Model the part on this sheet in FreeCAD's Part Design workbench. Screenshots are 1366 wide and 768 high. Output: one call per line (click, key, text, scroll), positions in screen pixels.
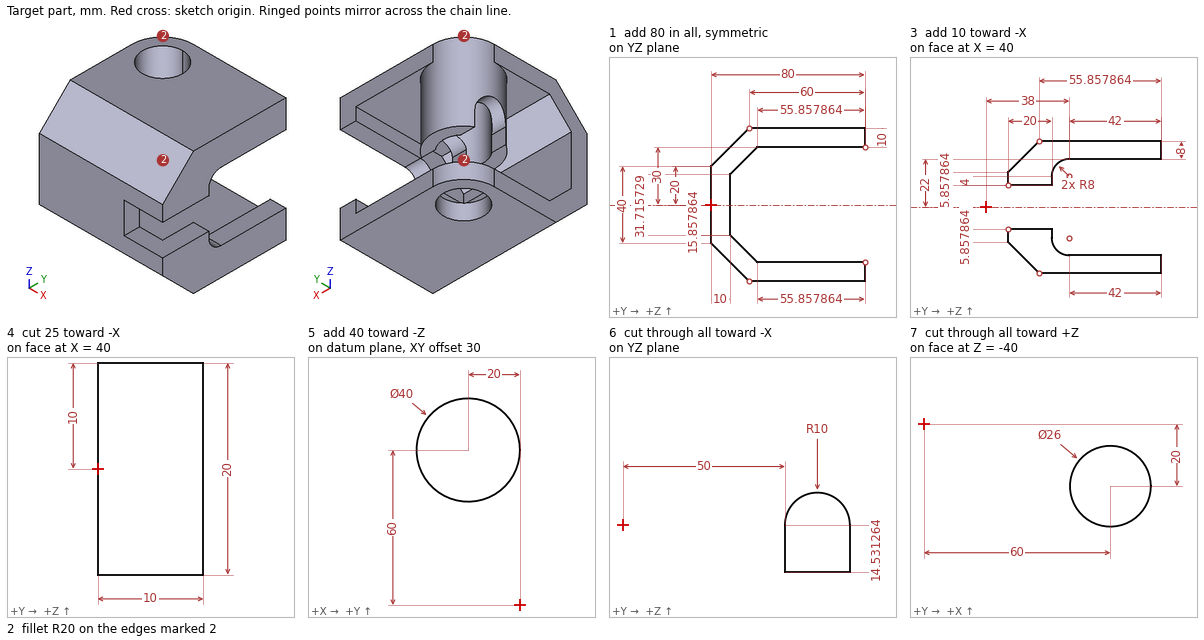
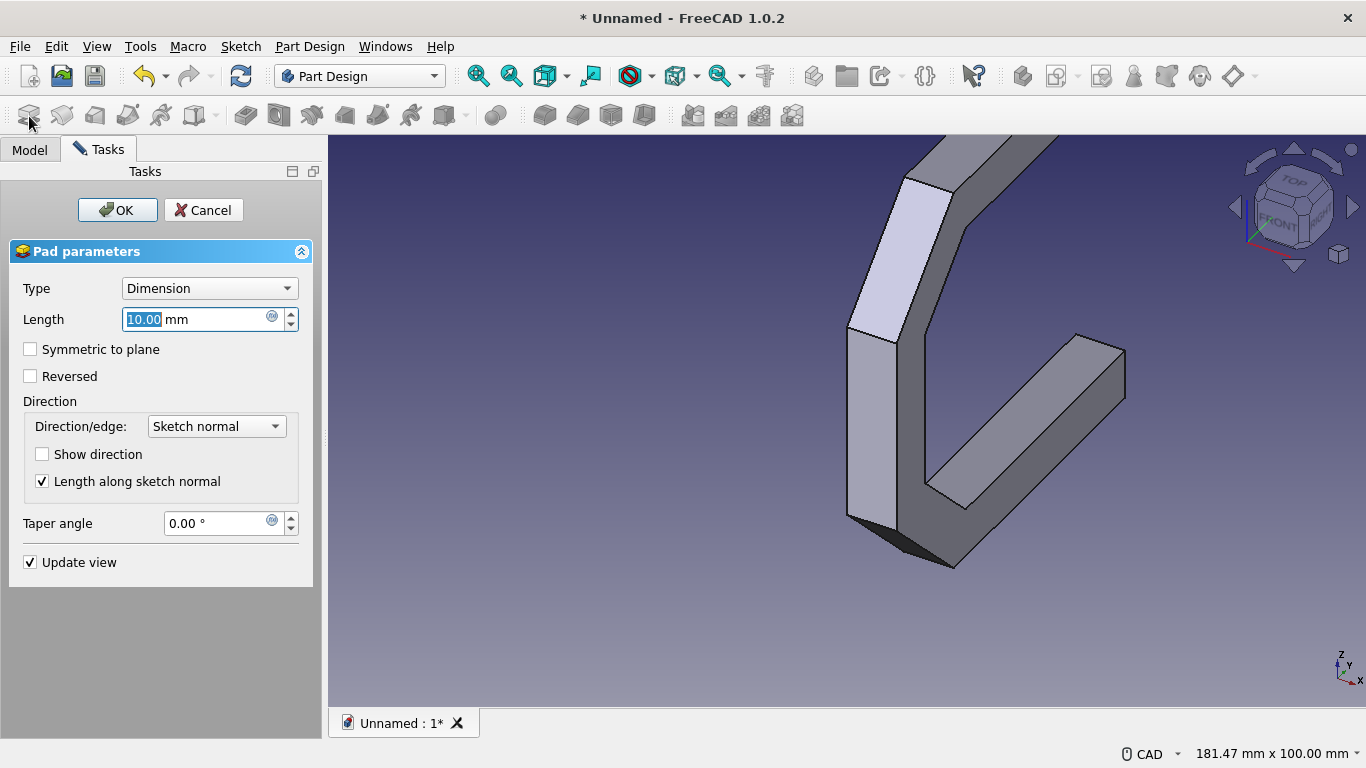
text(80)
key(Tab)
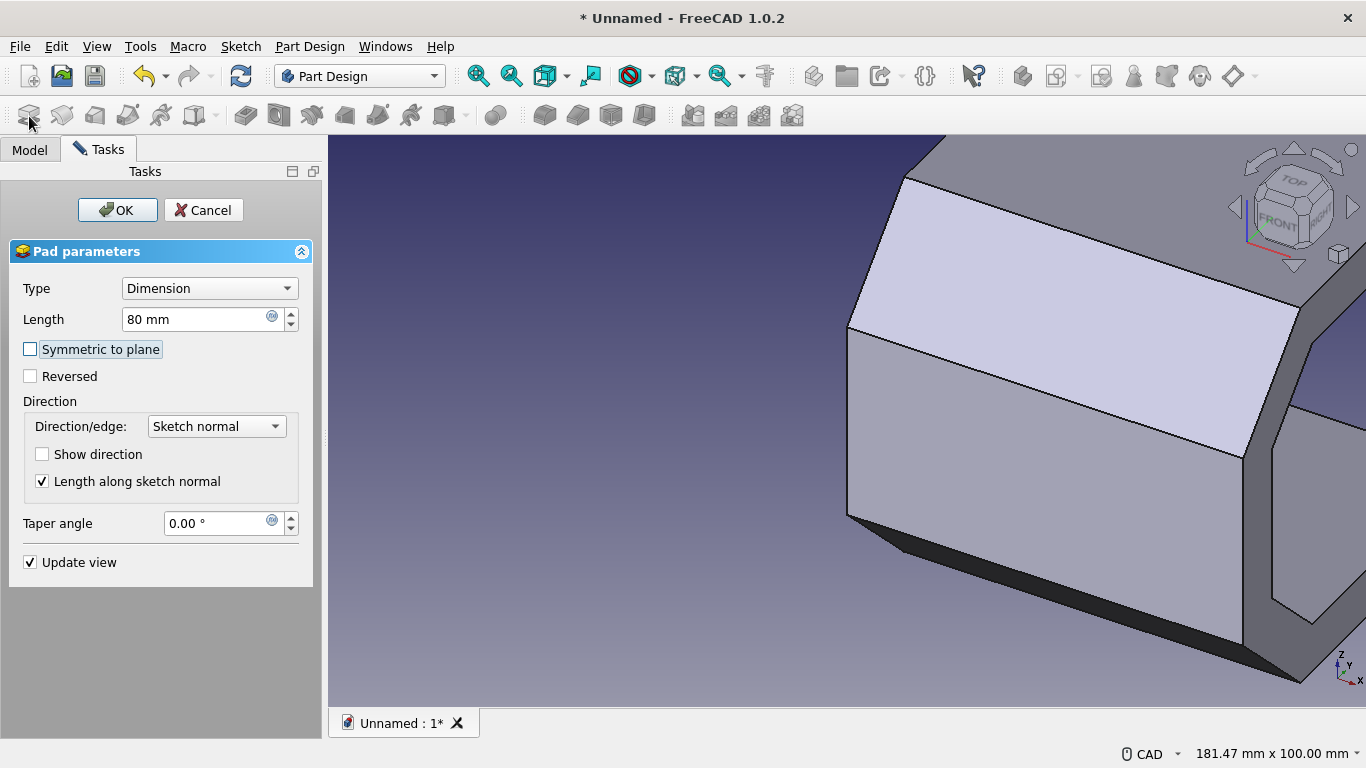
click(31, 349)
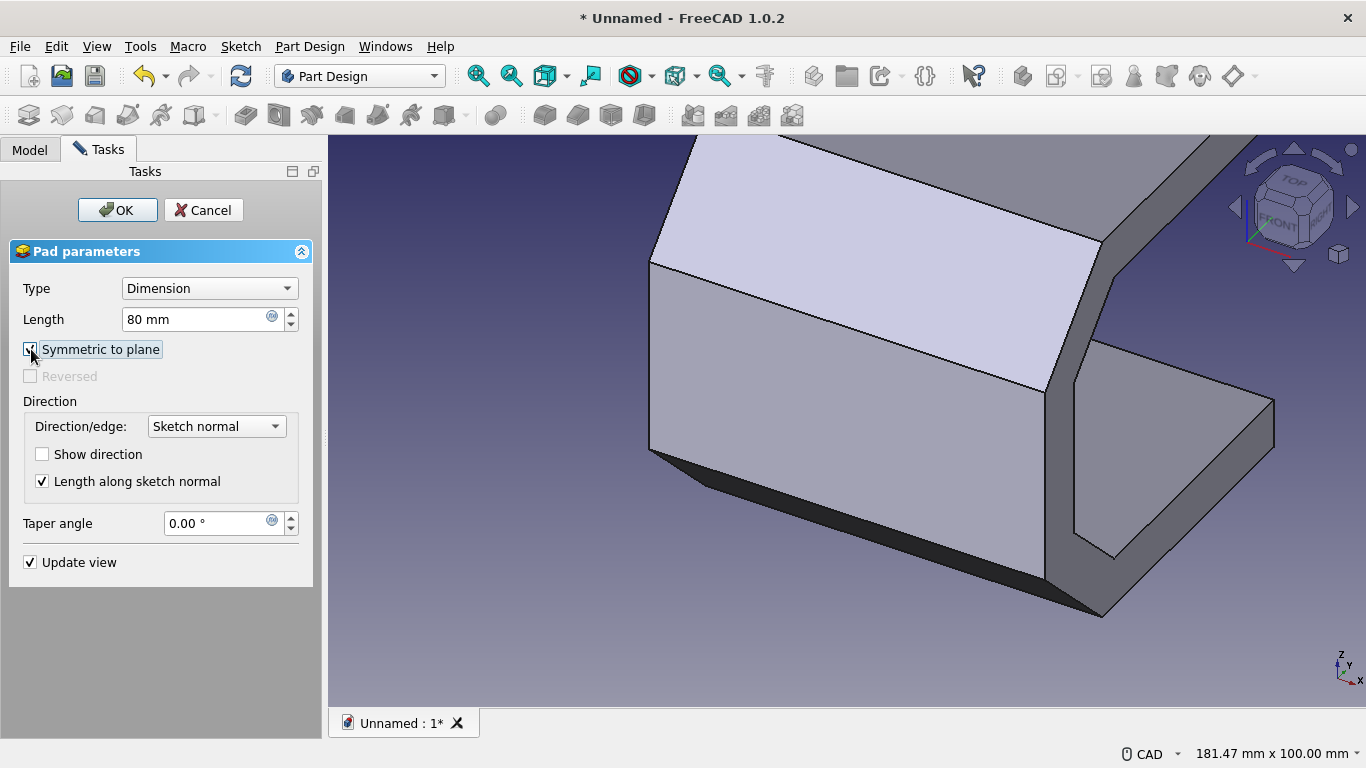
click(118, 210)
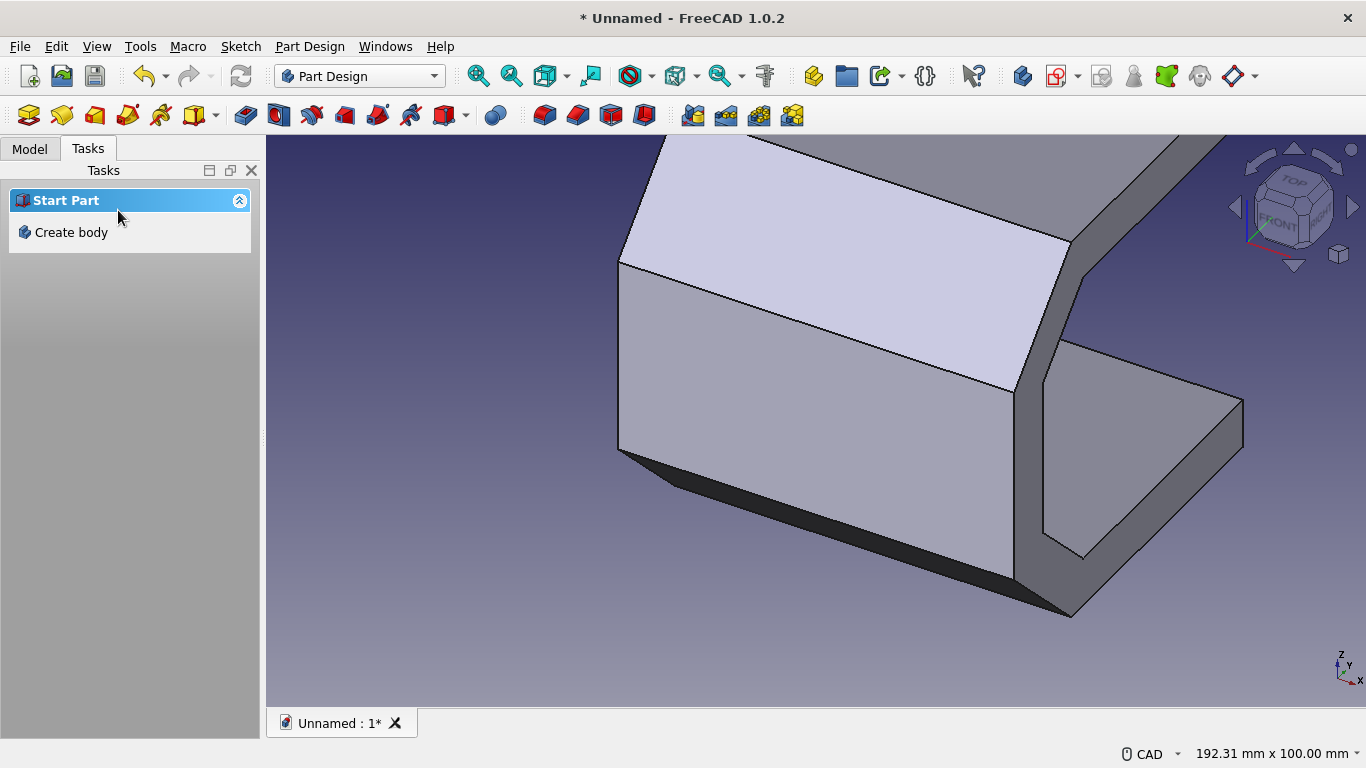
click(479, 76)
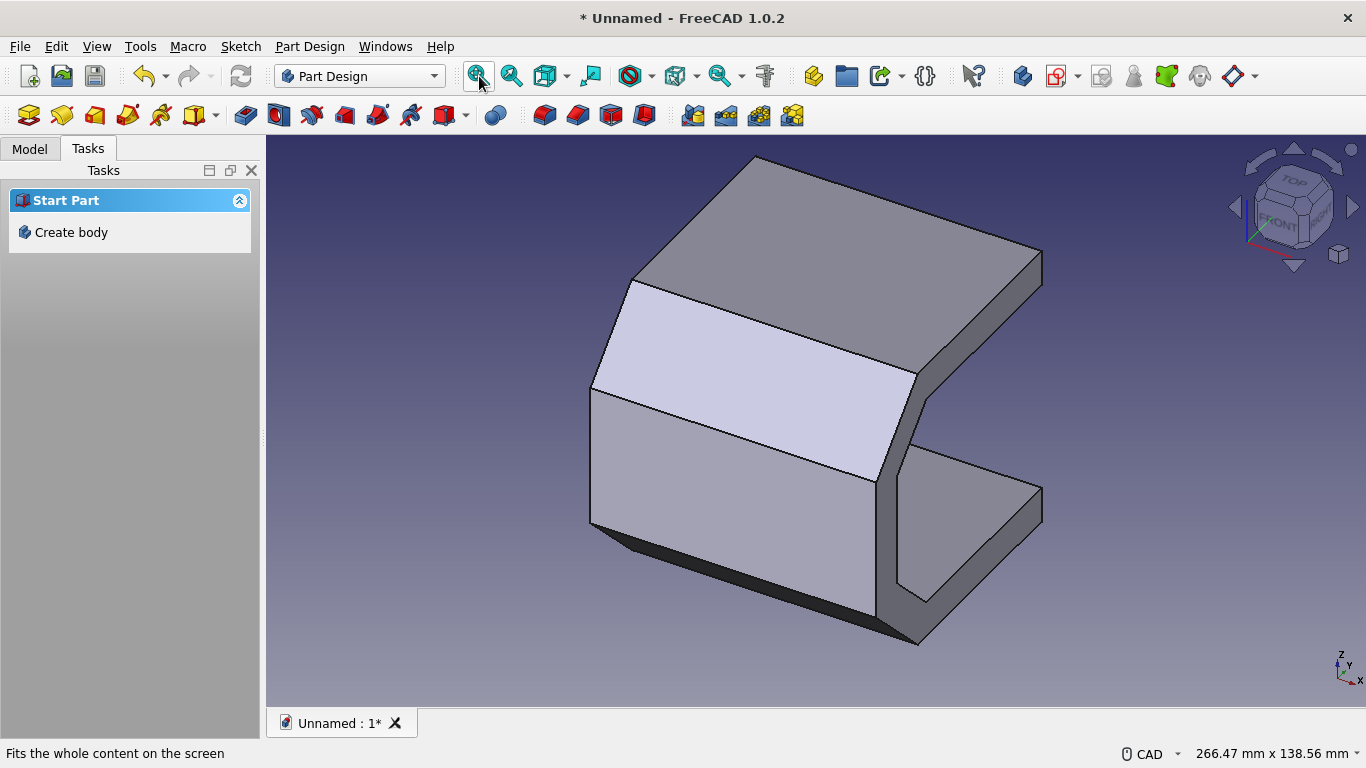
key(0)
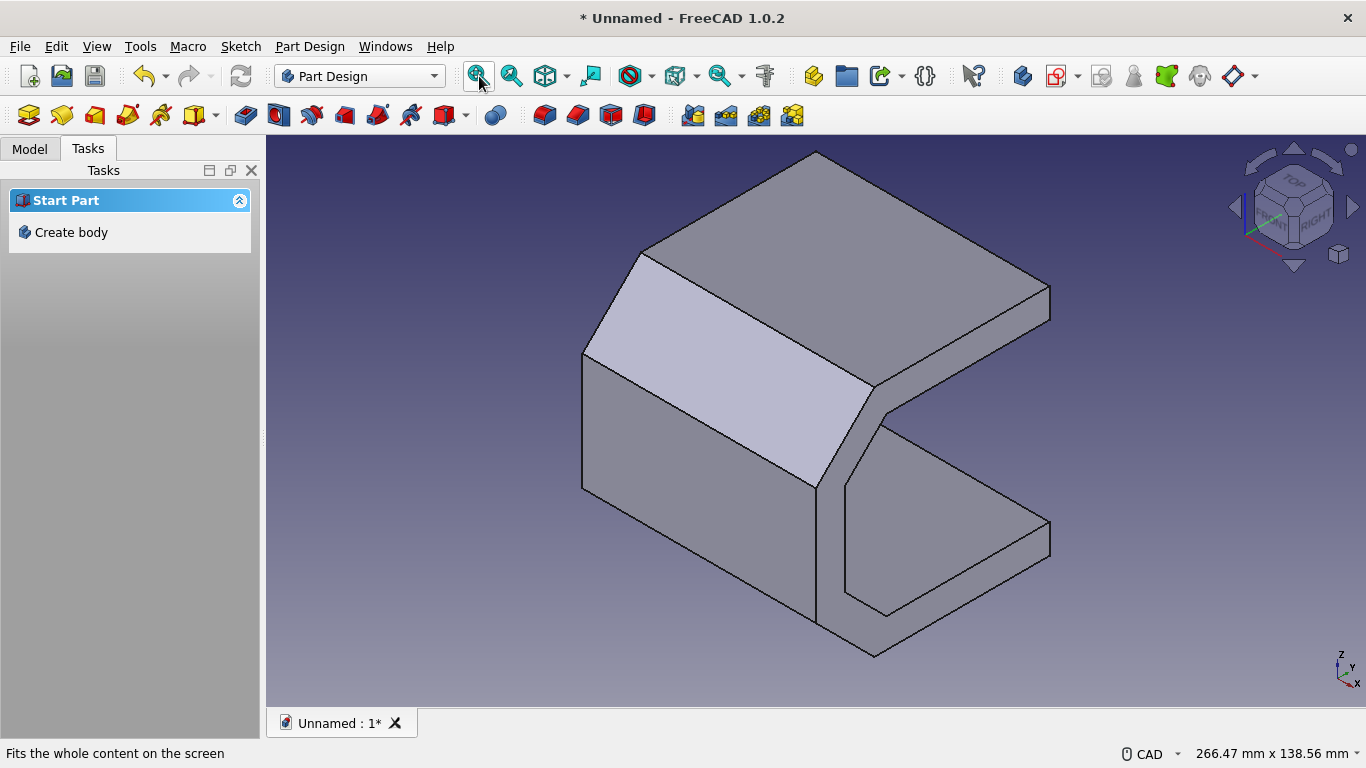
key(2)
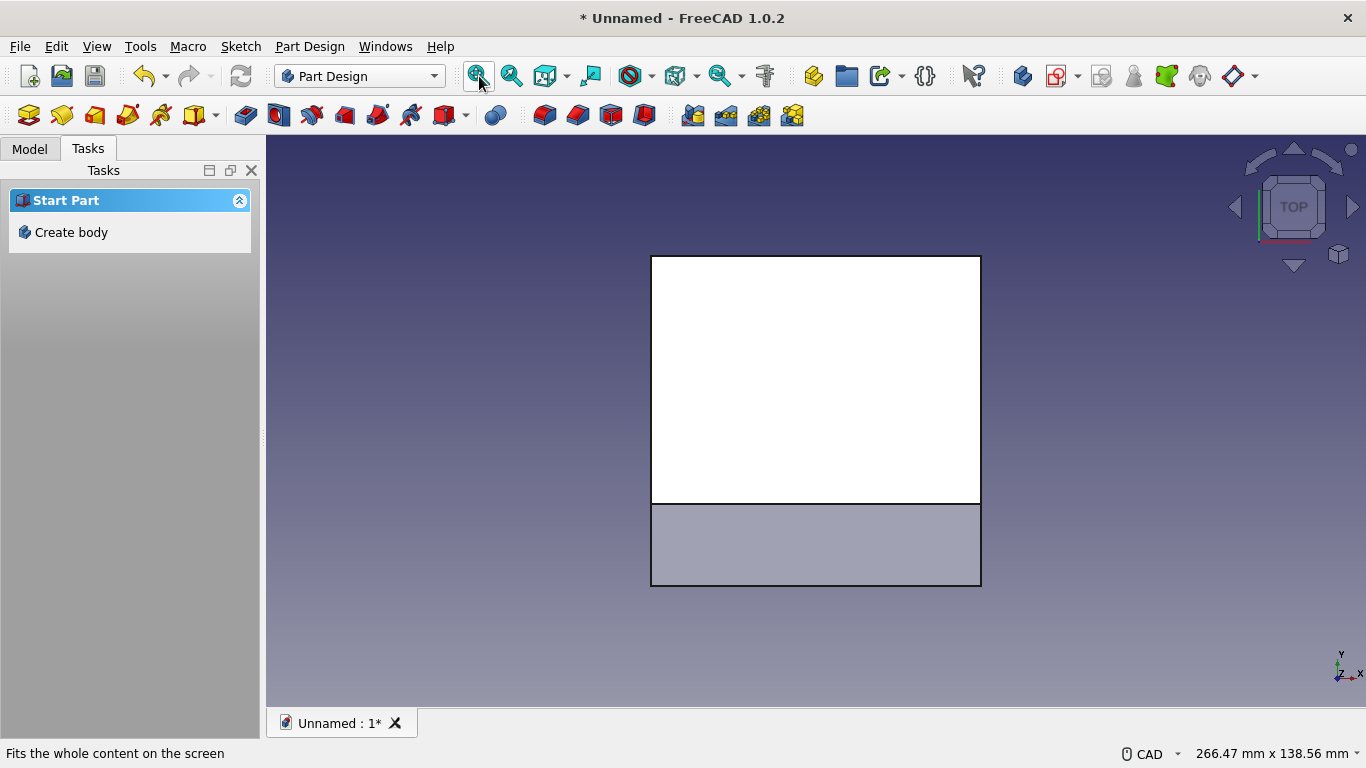
key(1)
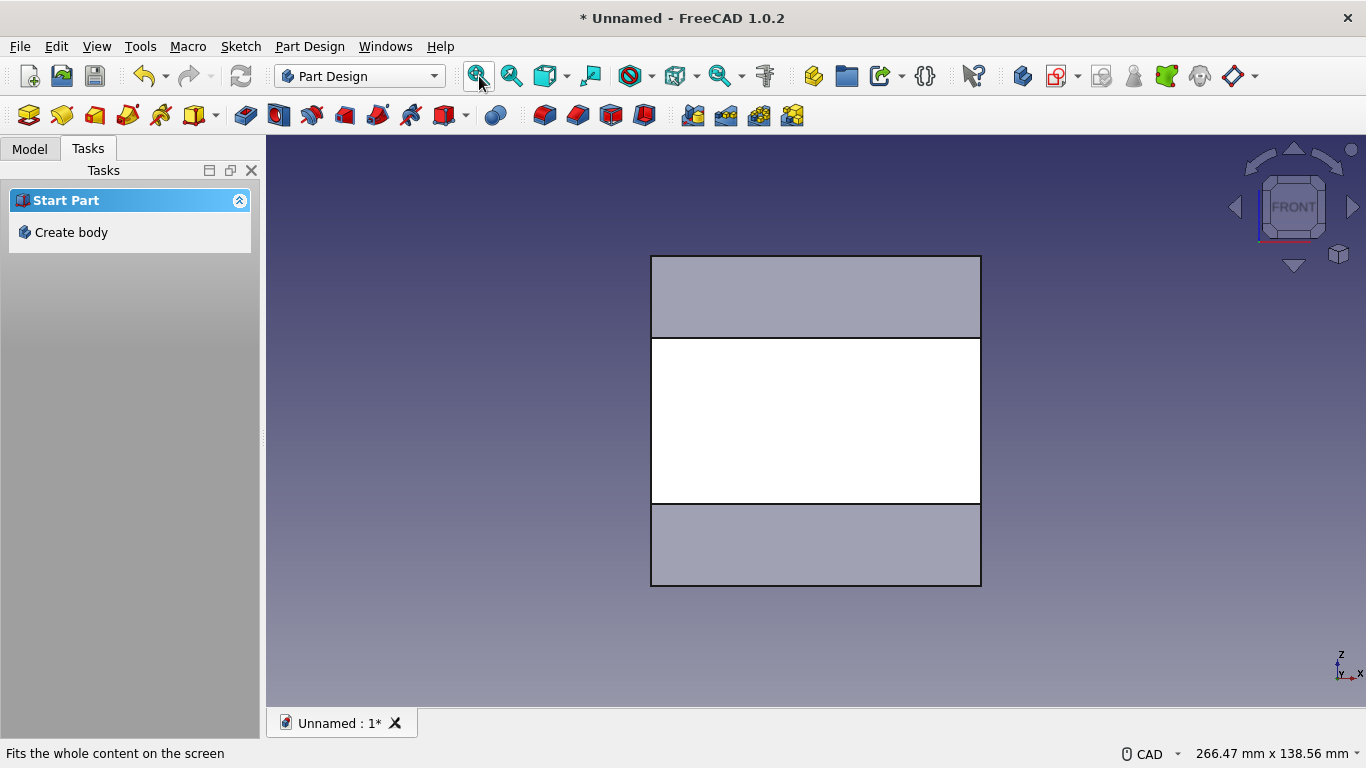
key(3)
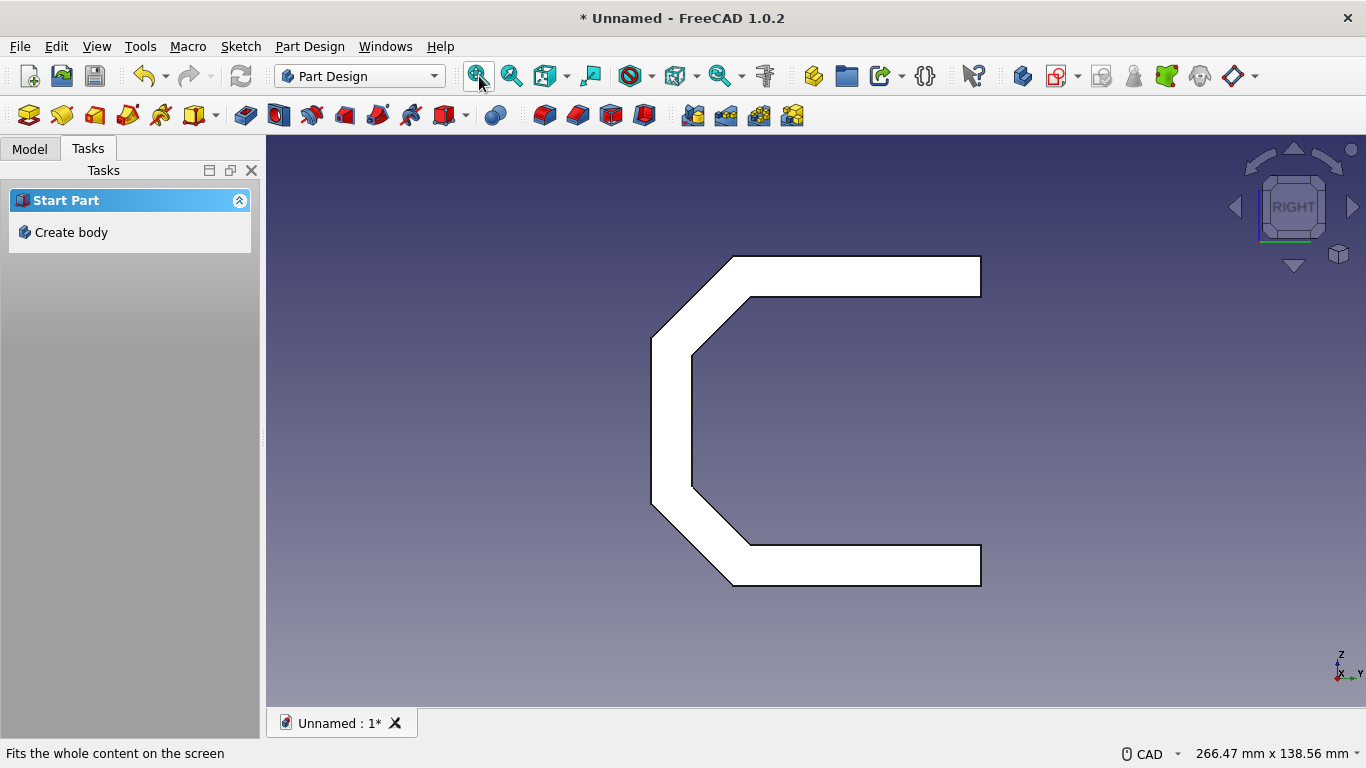
key(5)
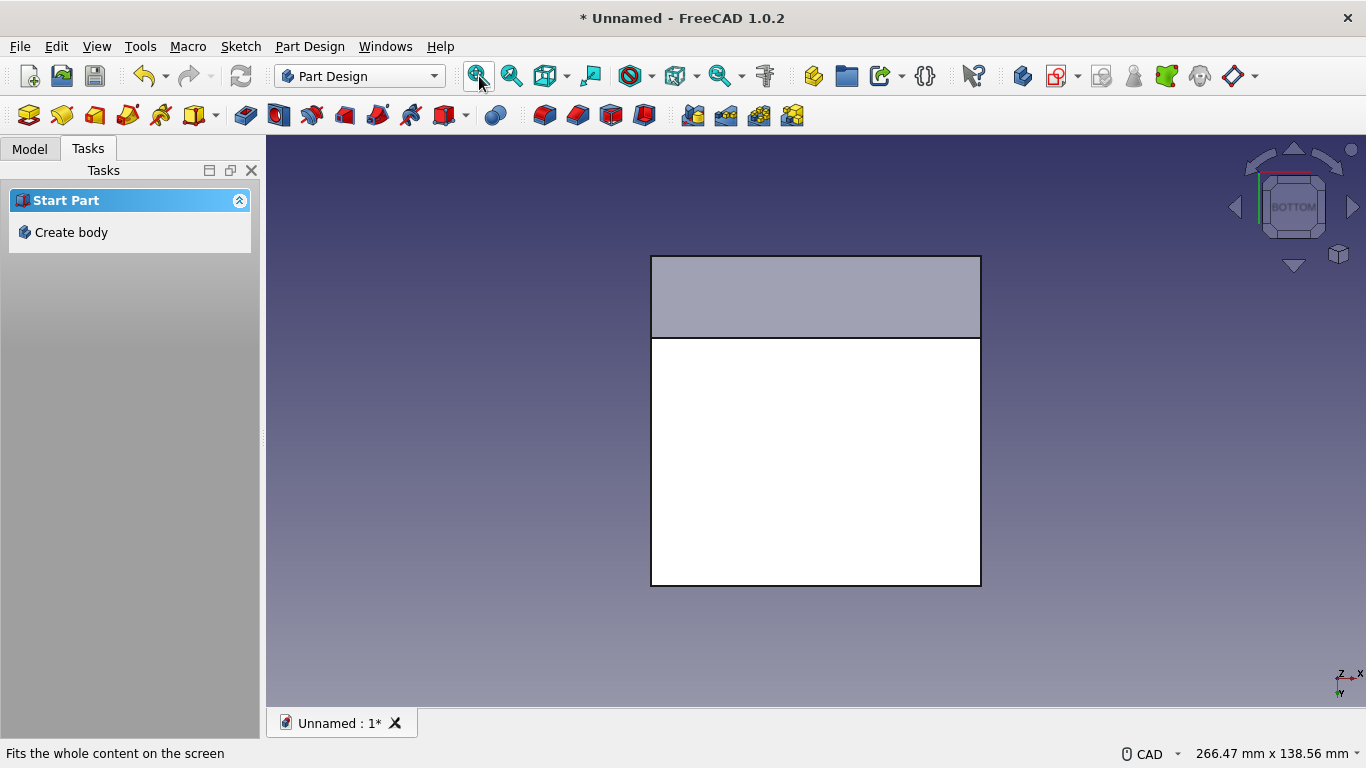
key(4)